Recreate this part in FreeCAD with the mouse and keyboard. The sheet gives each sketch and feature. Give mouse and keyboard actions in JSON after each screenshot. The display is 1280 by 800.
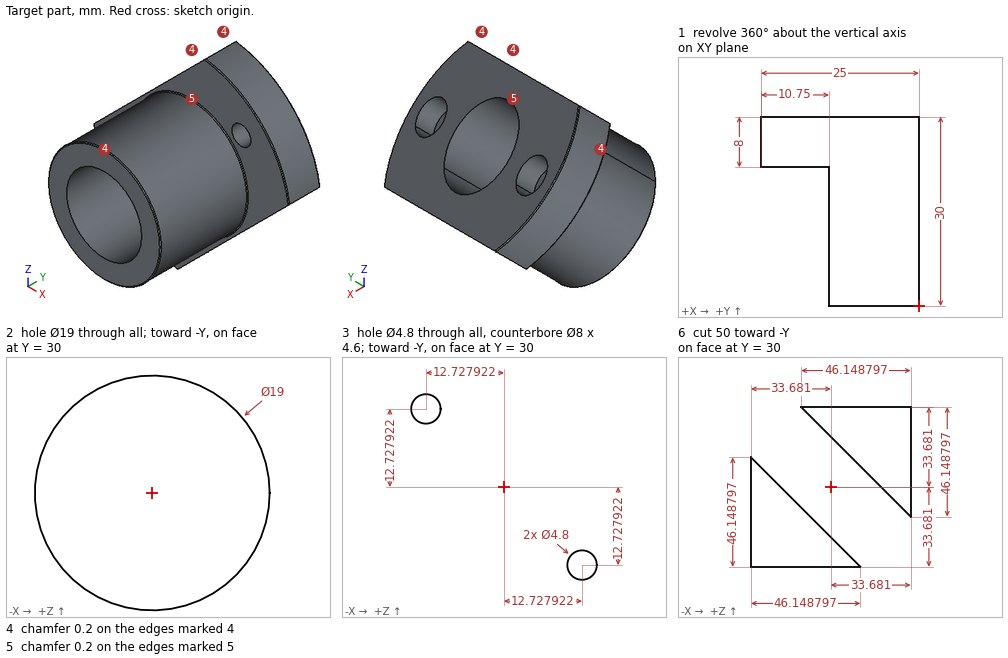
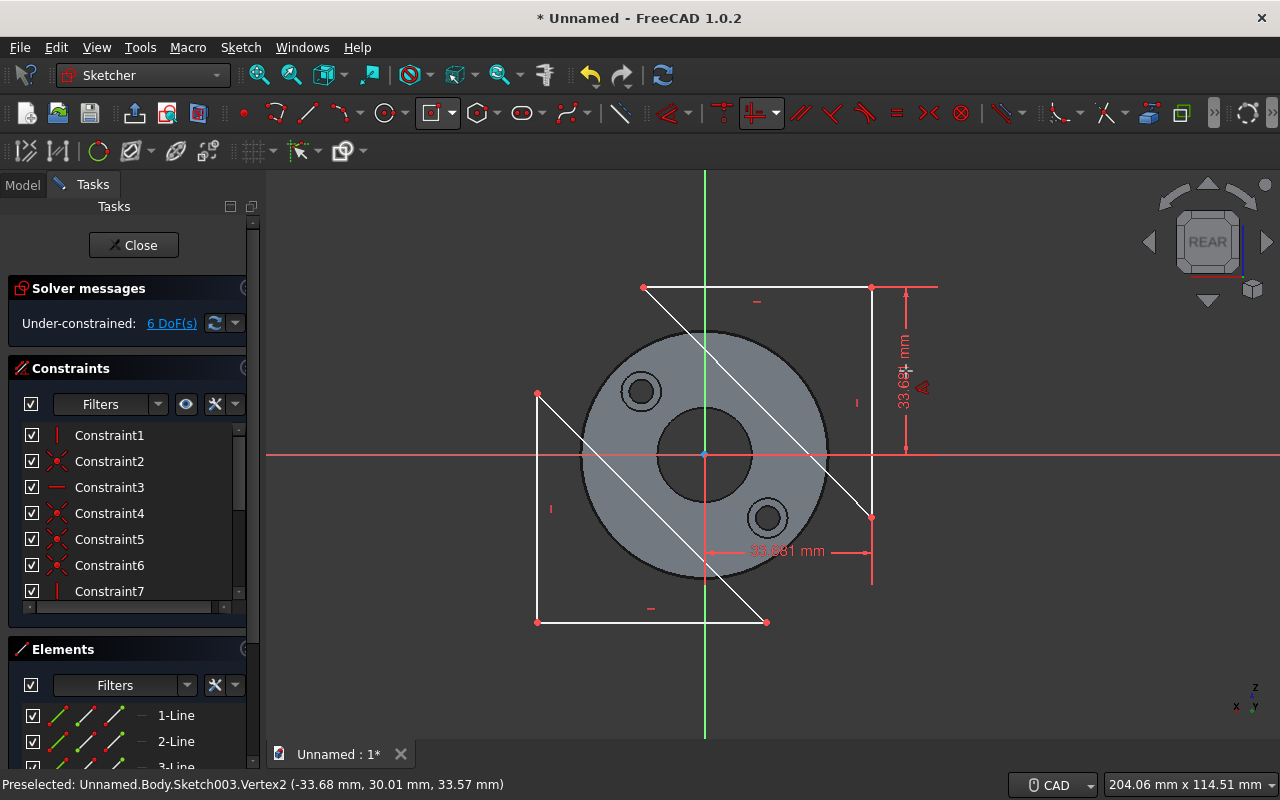
{"action": "left_click", "coordinate": [766, 623]}
{"action": "left_click", "coordinate": [800, 500]}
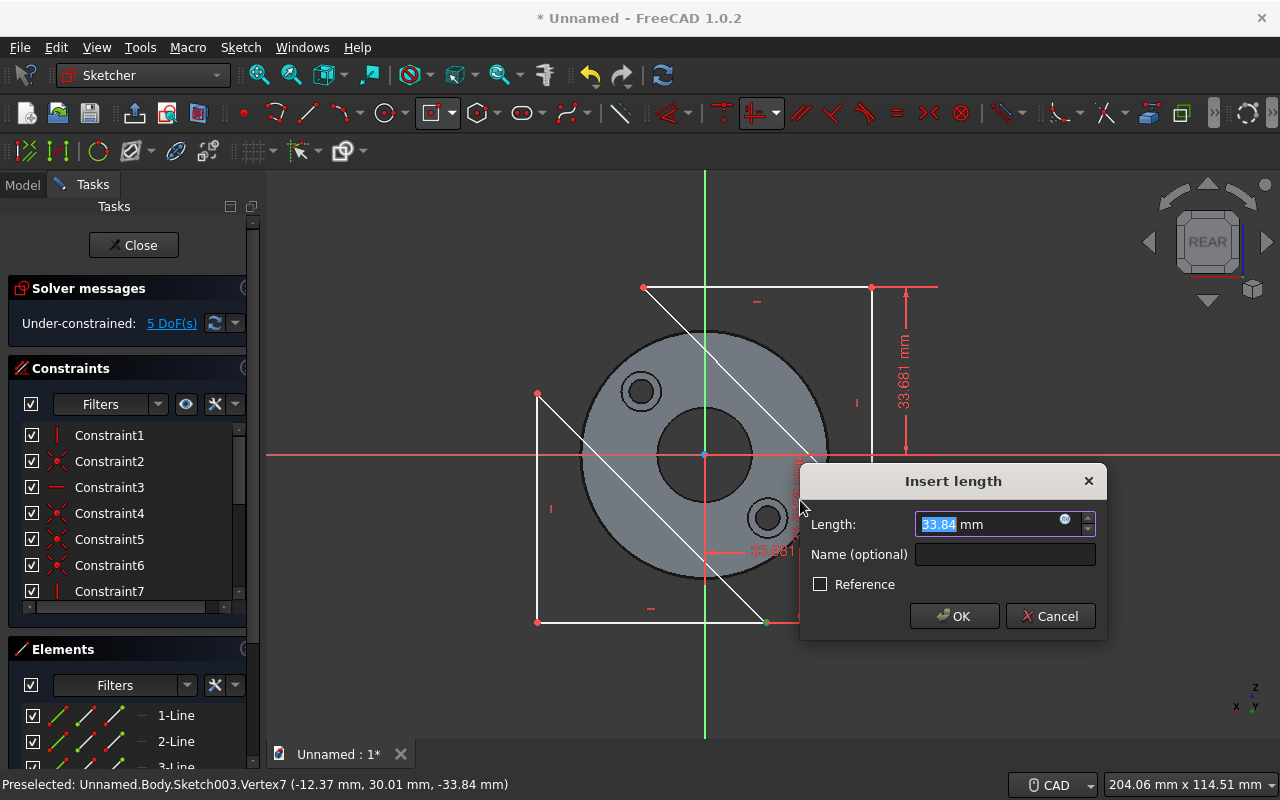
{"action": "type", "text": "33.681"}
{"action": "key", "text": "Return"}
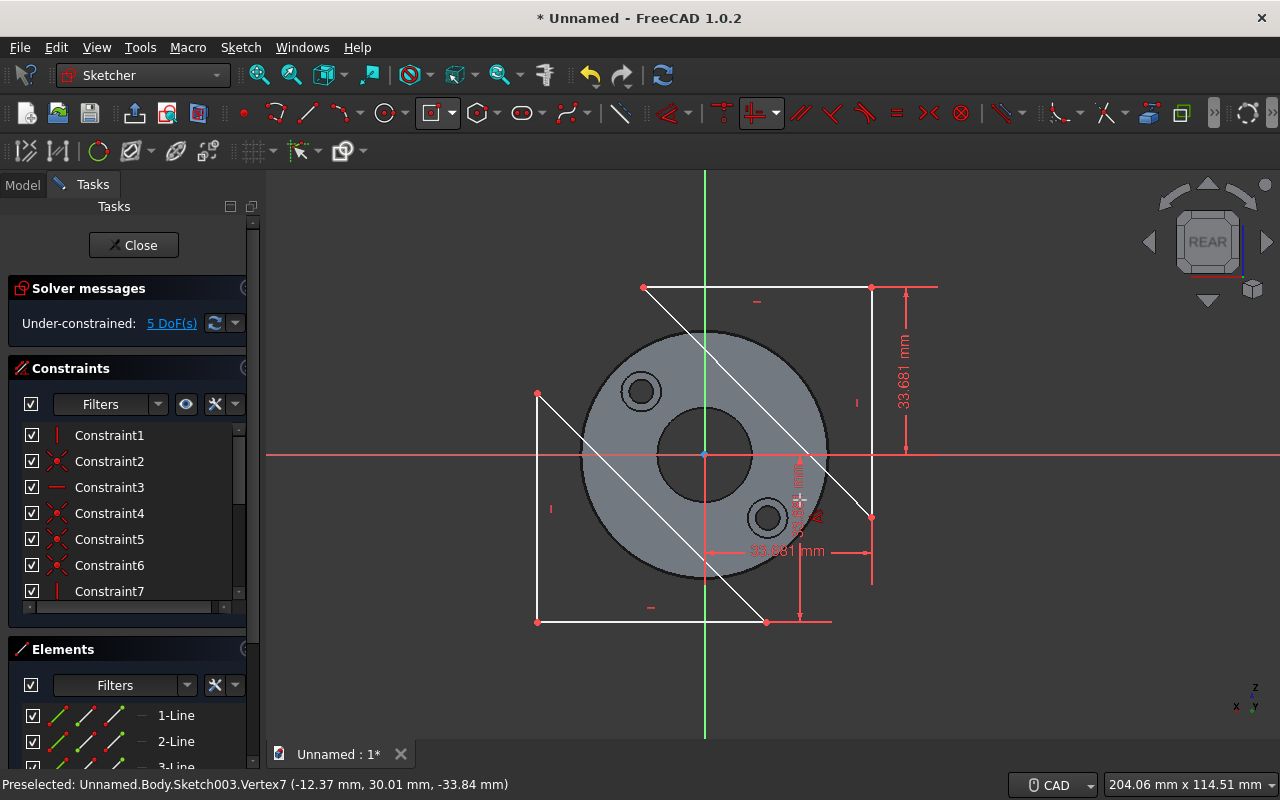
{"action": "left_click", "coordinate": [537, 394]}
{"action": "left_click", "coordinate": [621, 360]}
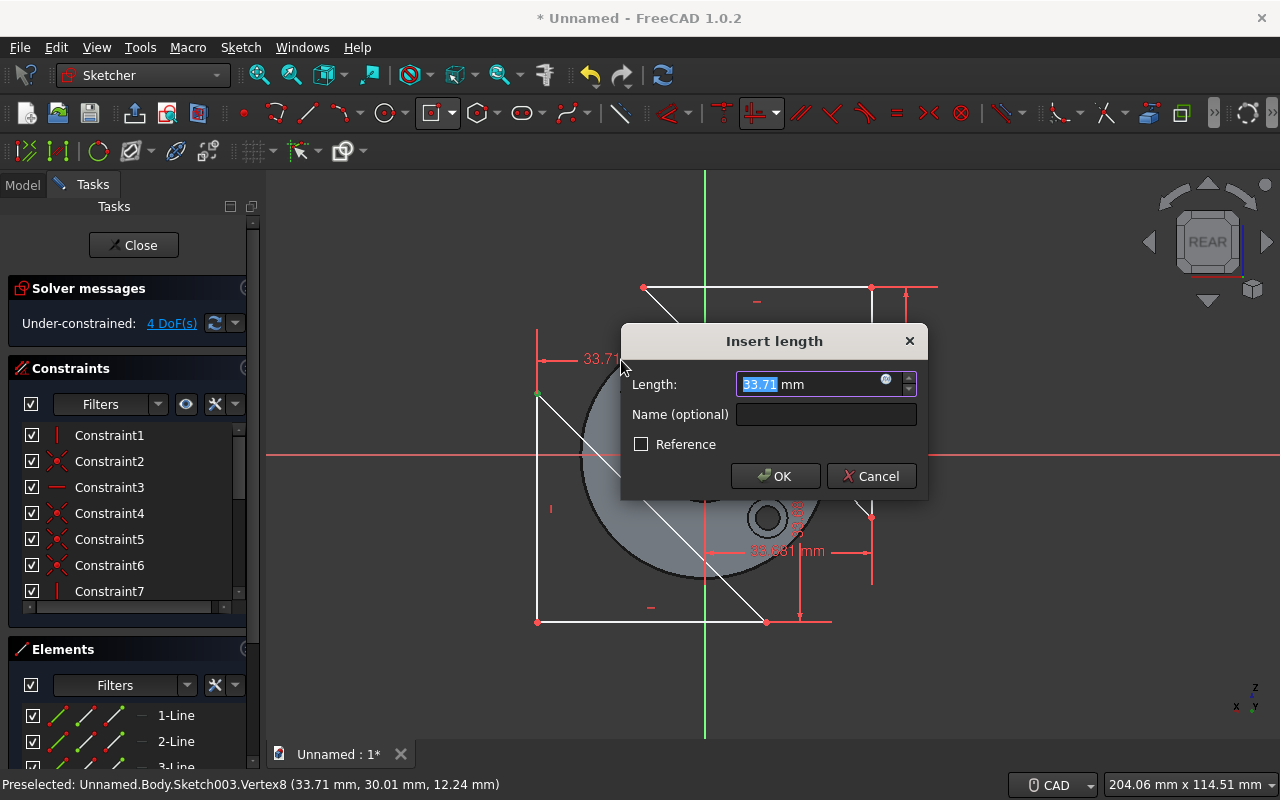
{"action": "type", "text": "33.681"}
{"action": "key", "text": "Return"}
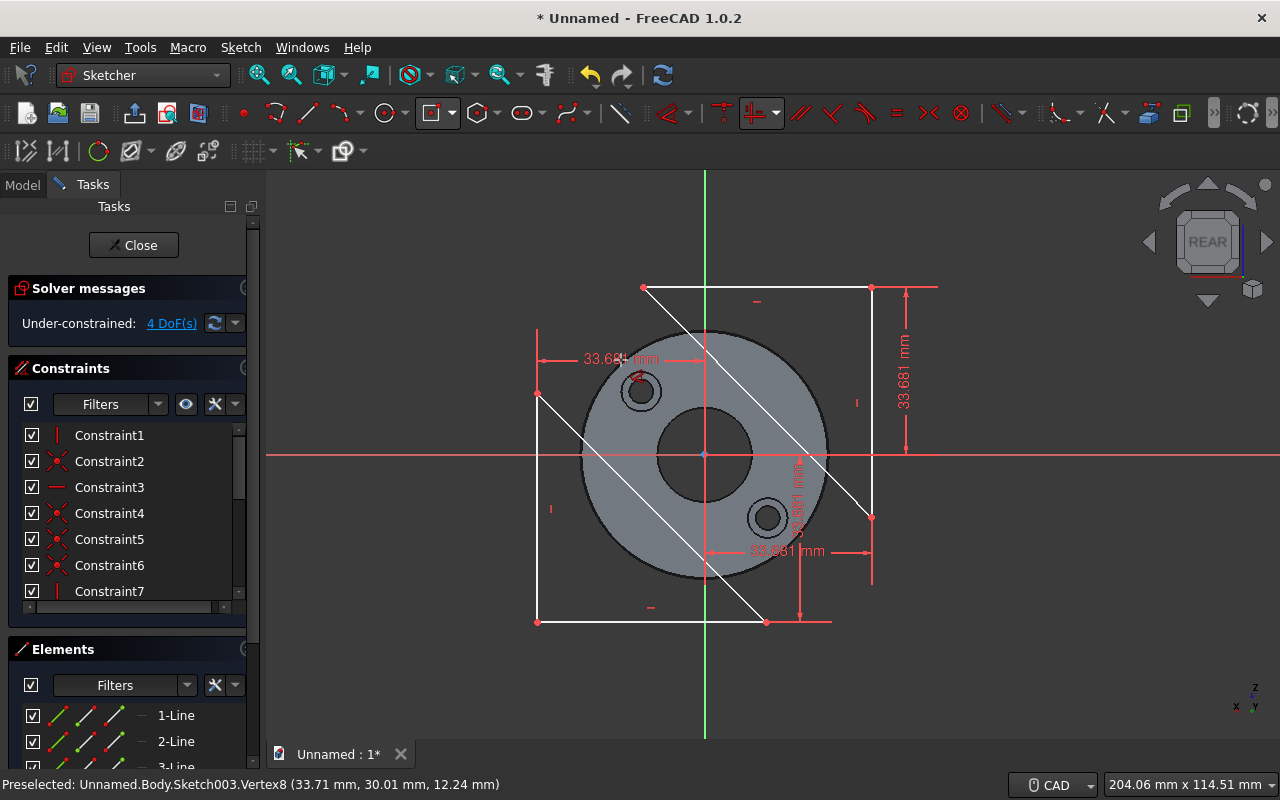
{"action": "left_click", "coordinate": [872, 357]}
{"action": "left_click", "coordinate": [906, 403]}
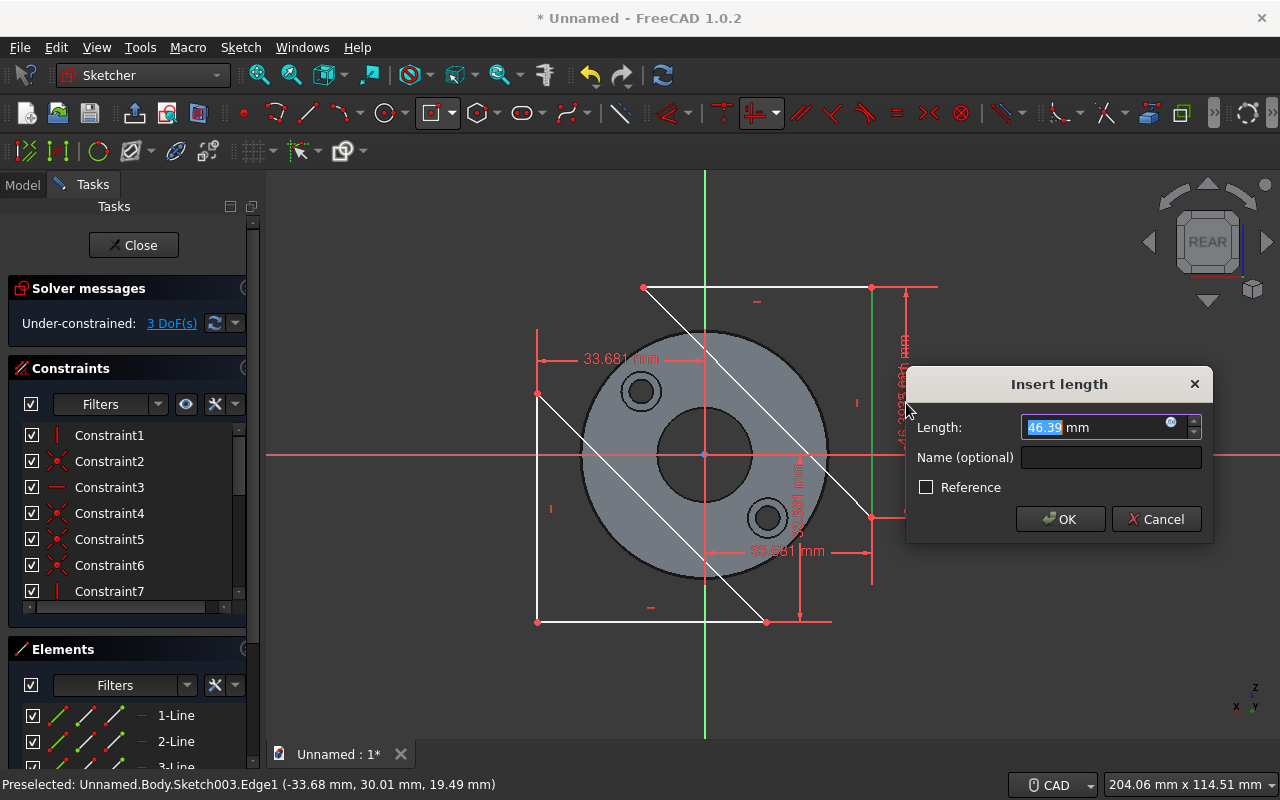
{"action": "type", "text": "46.148797"}
{"action": "key", "text": "Return"}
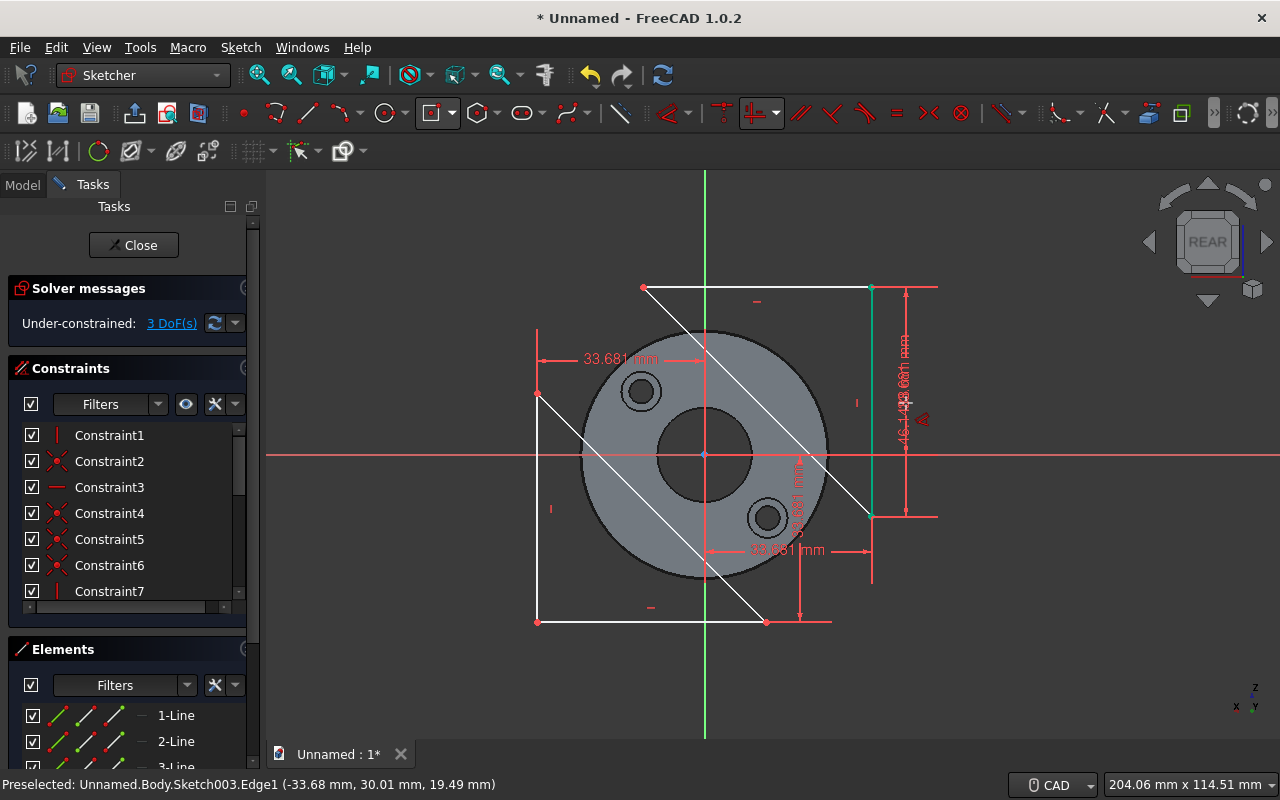
{"action": "left_click", "coordinate": [803, 287]}
{"action": "left_click", "coordinate": [757, 253]}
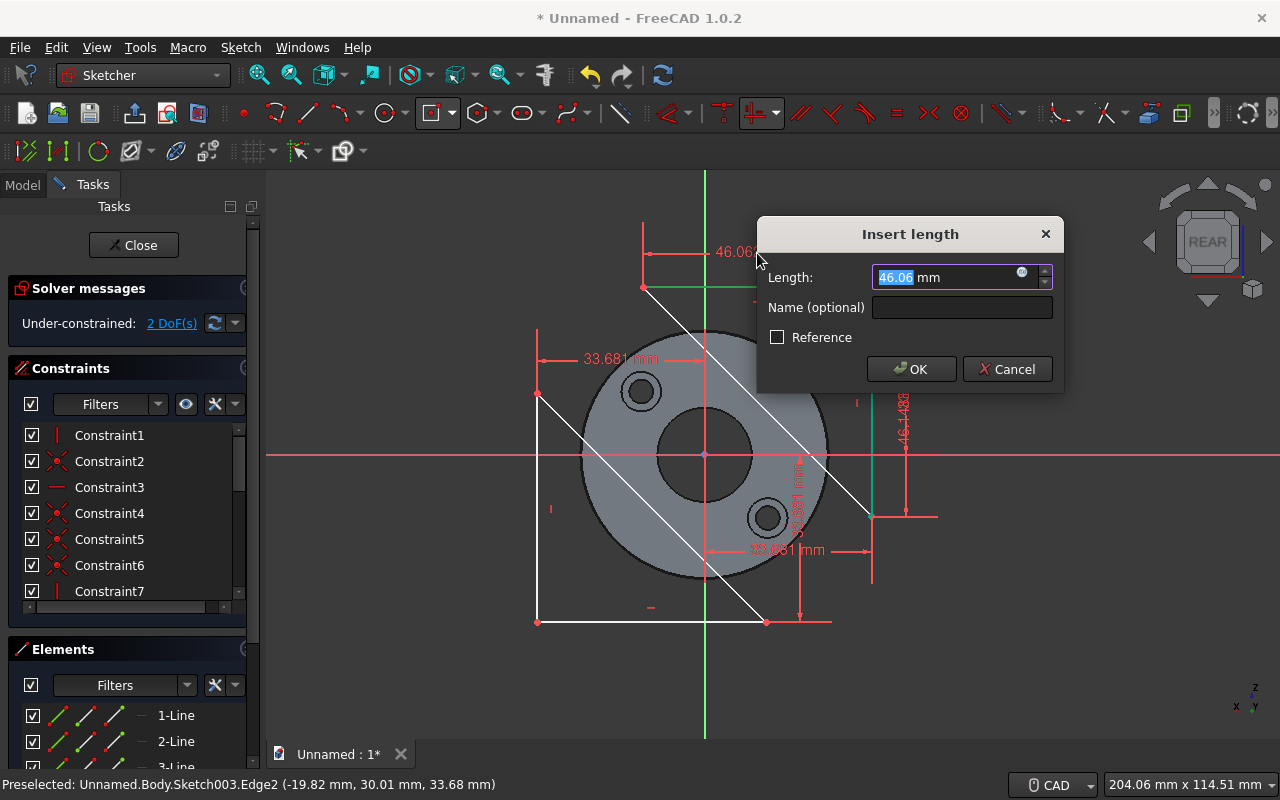
{"action": "type", "text": "46.148797"}
{"action": "key", "text": "Return"}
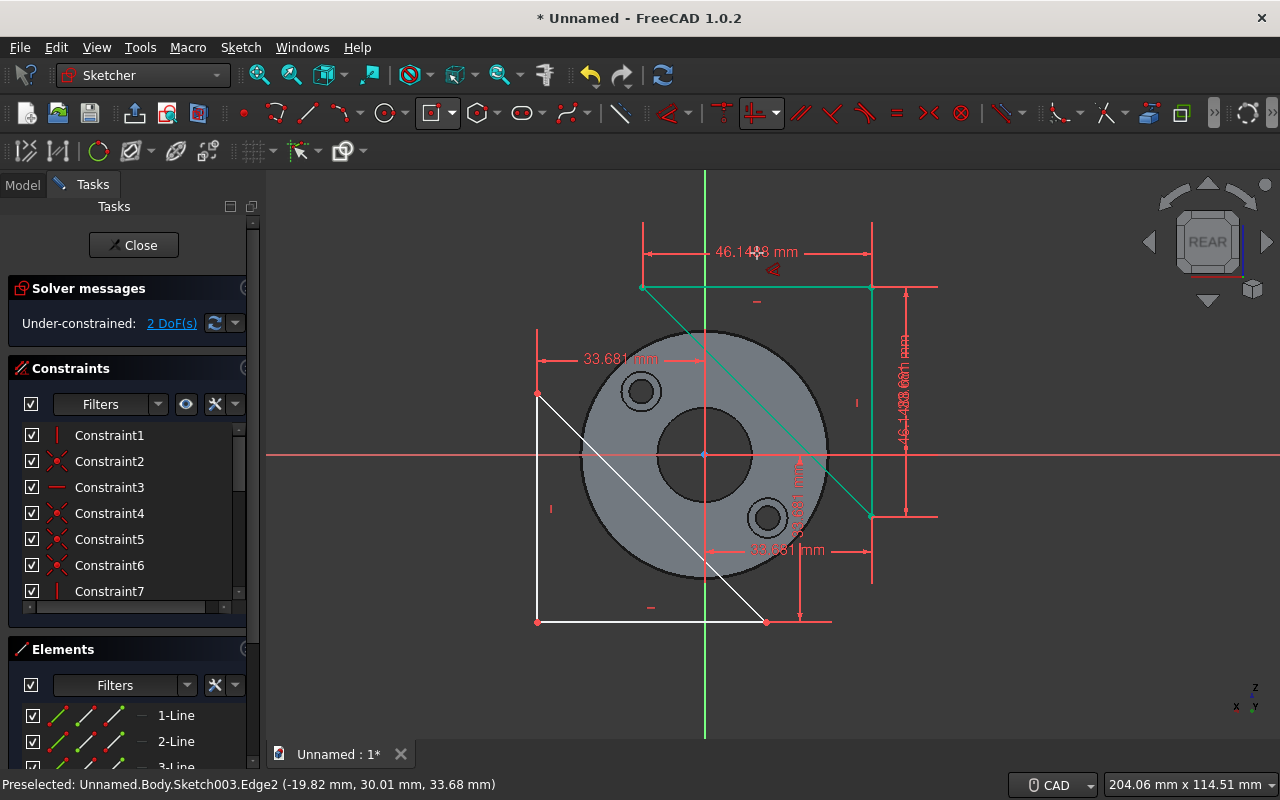
{"action": "left_click", "coordinate": [537, 554]}
{"action": "left_click", "coordinate": [503, 508]}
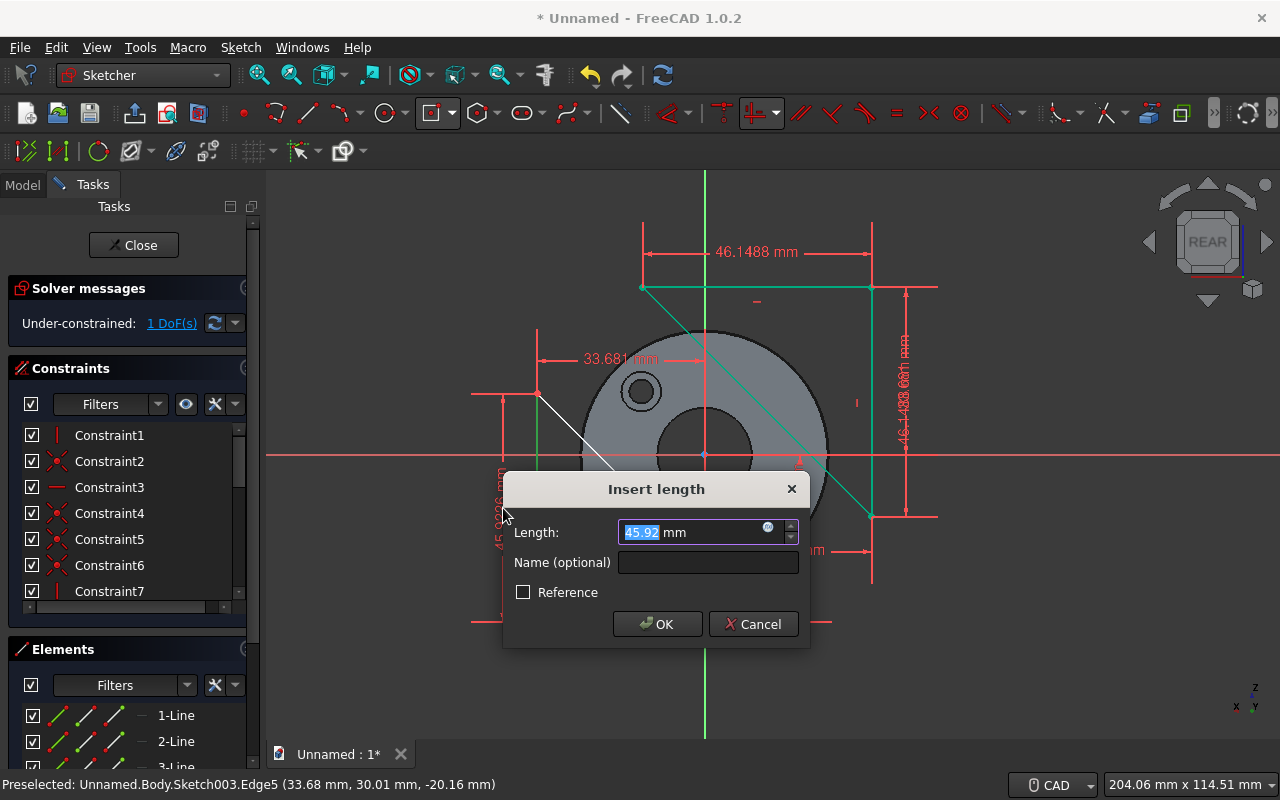
{"action": "type", "text": "46.148797"}
{"action": "key", "text": "Return"}